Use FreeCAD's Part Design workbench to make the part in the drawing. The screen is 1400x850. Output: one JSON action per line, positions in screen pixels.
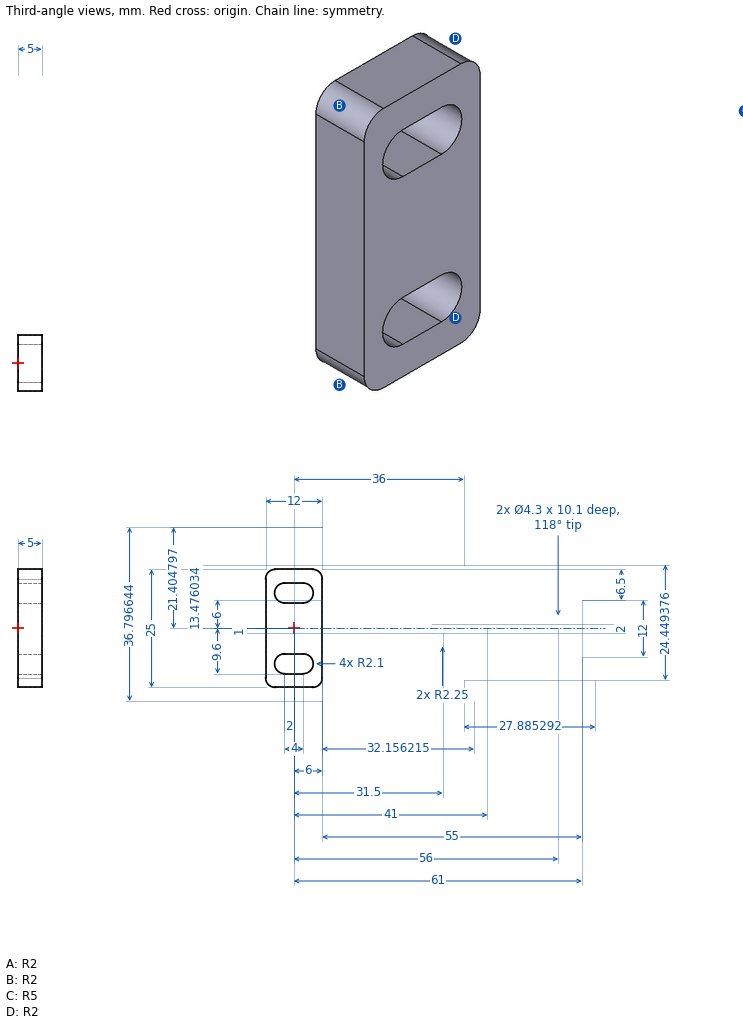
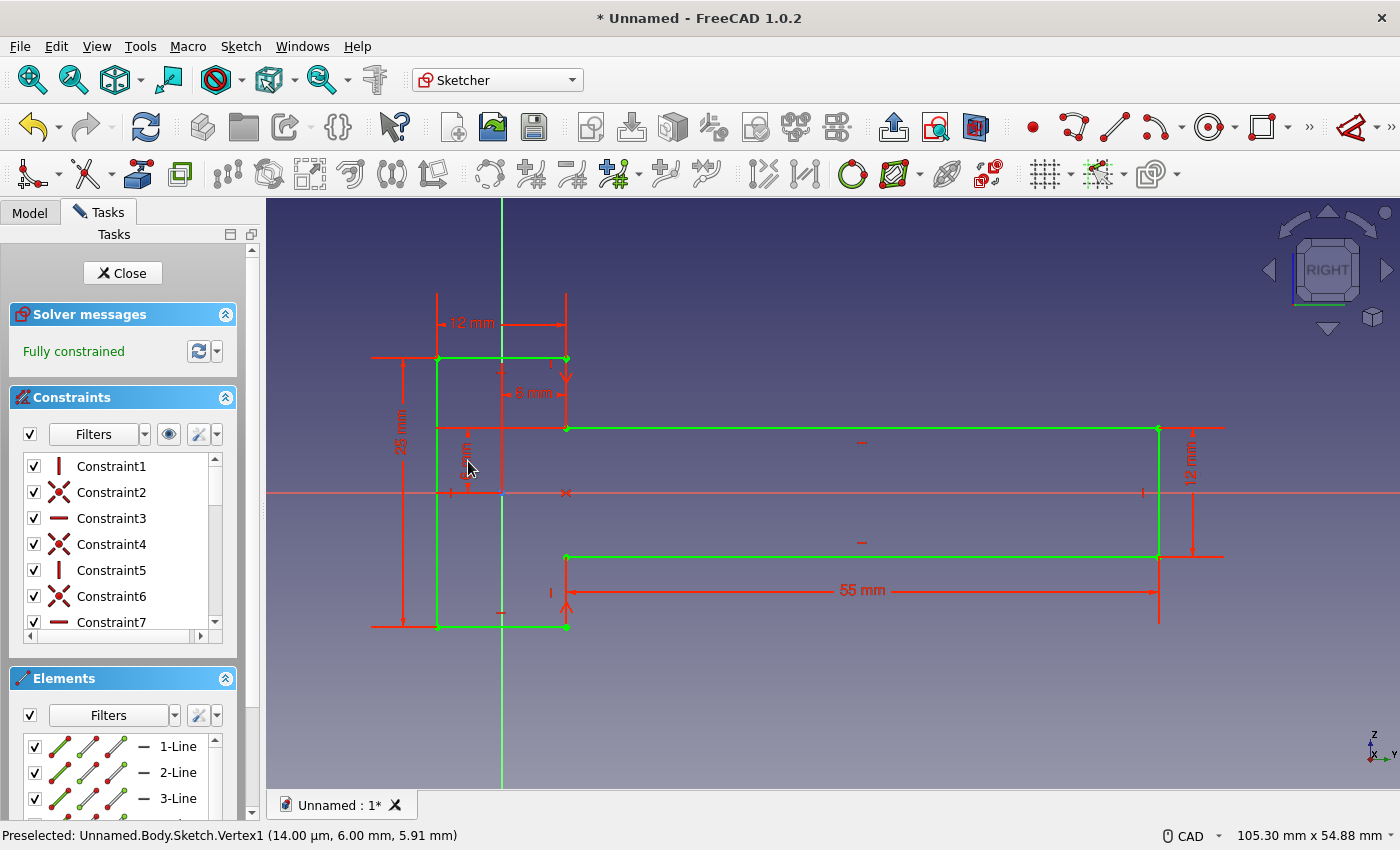
{"action": "left_click", "coordinate": [123, 273]}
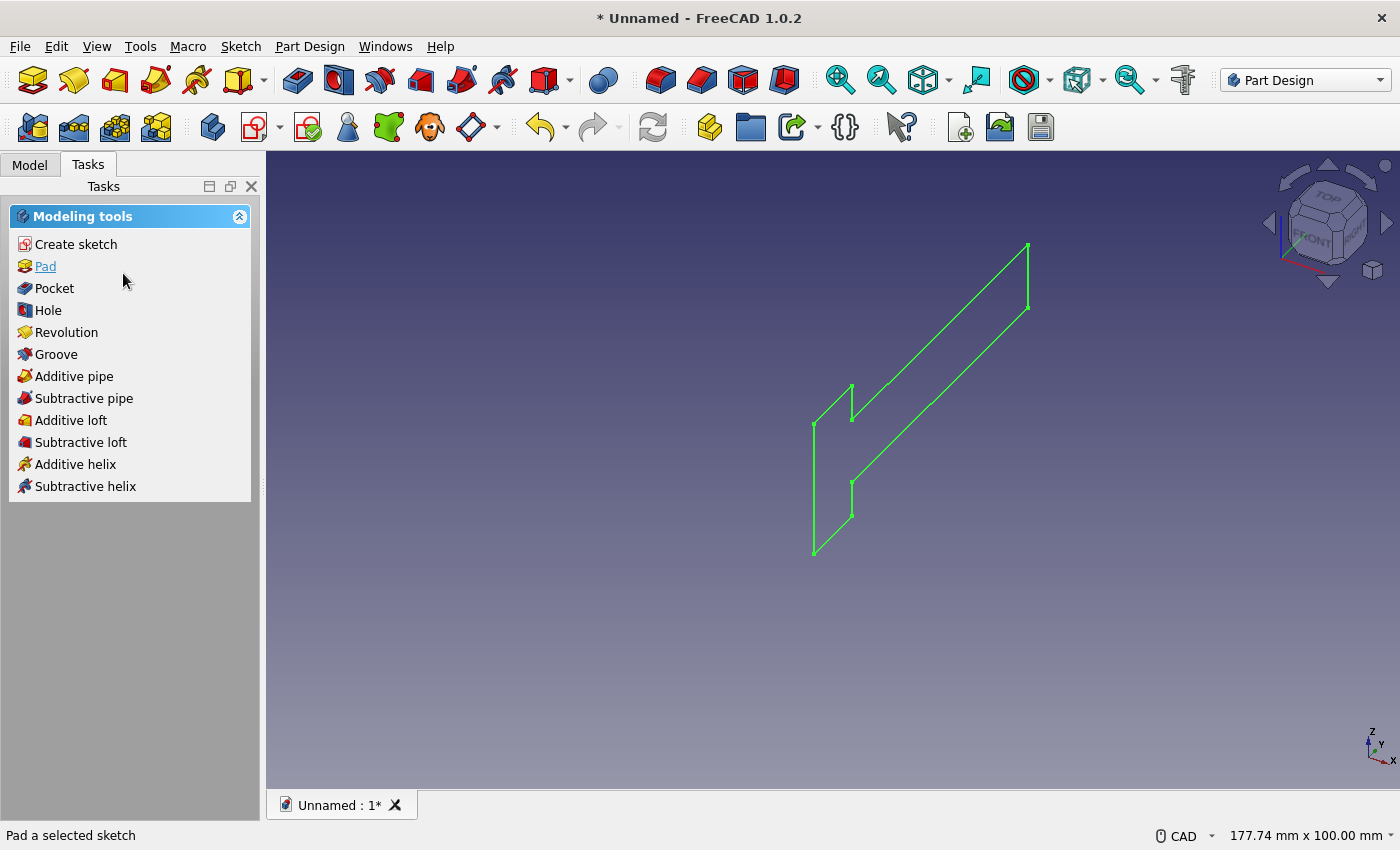
{"action": "left_click", "coordinate": [33, 80]}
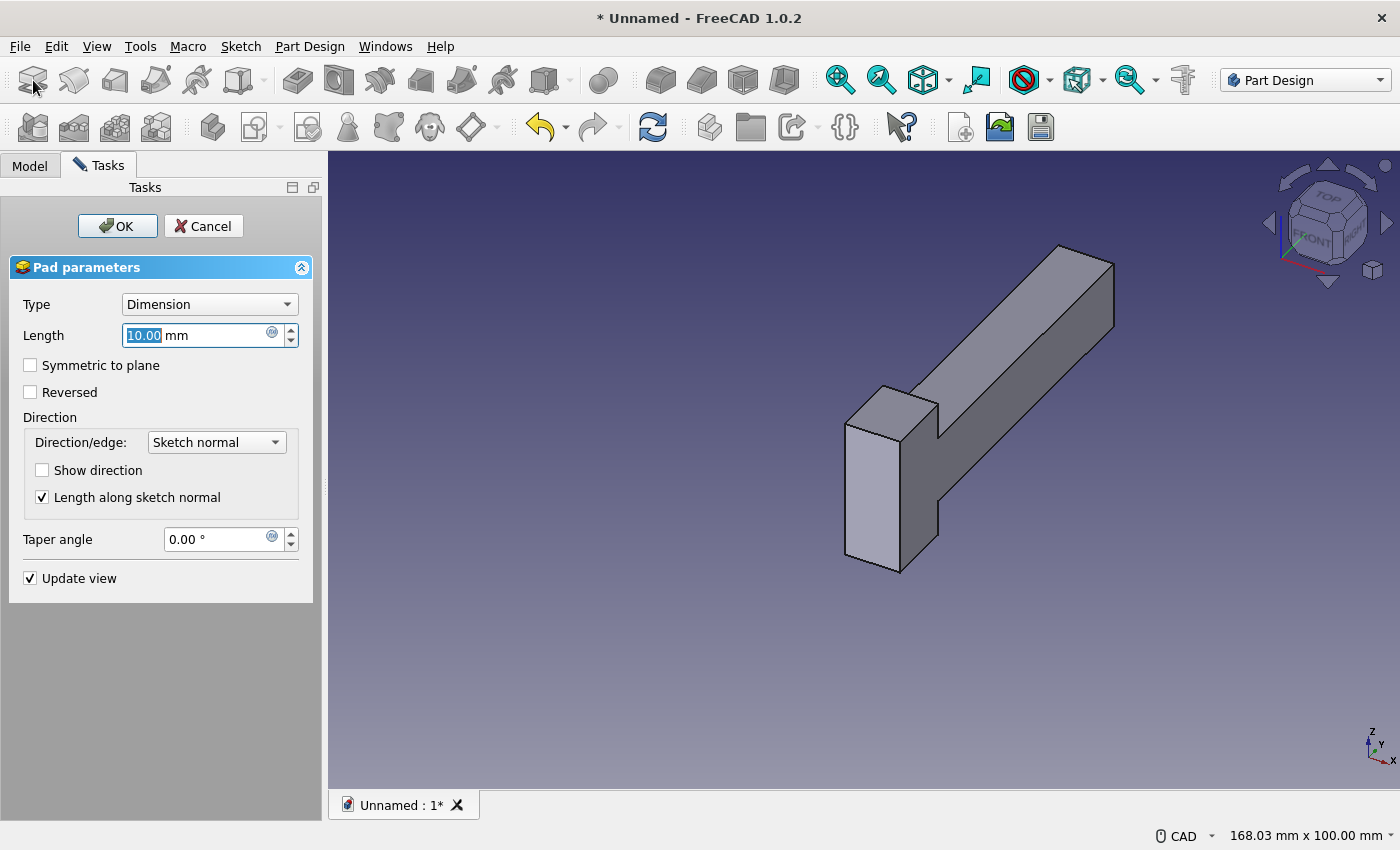
{"action": "type", "text": "5"}
{"action": "key", "text": "Tab"}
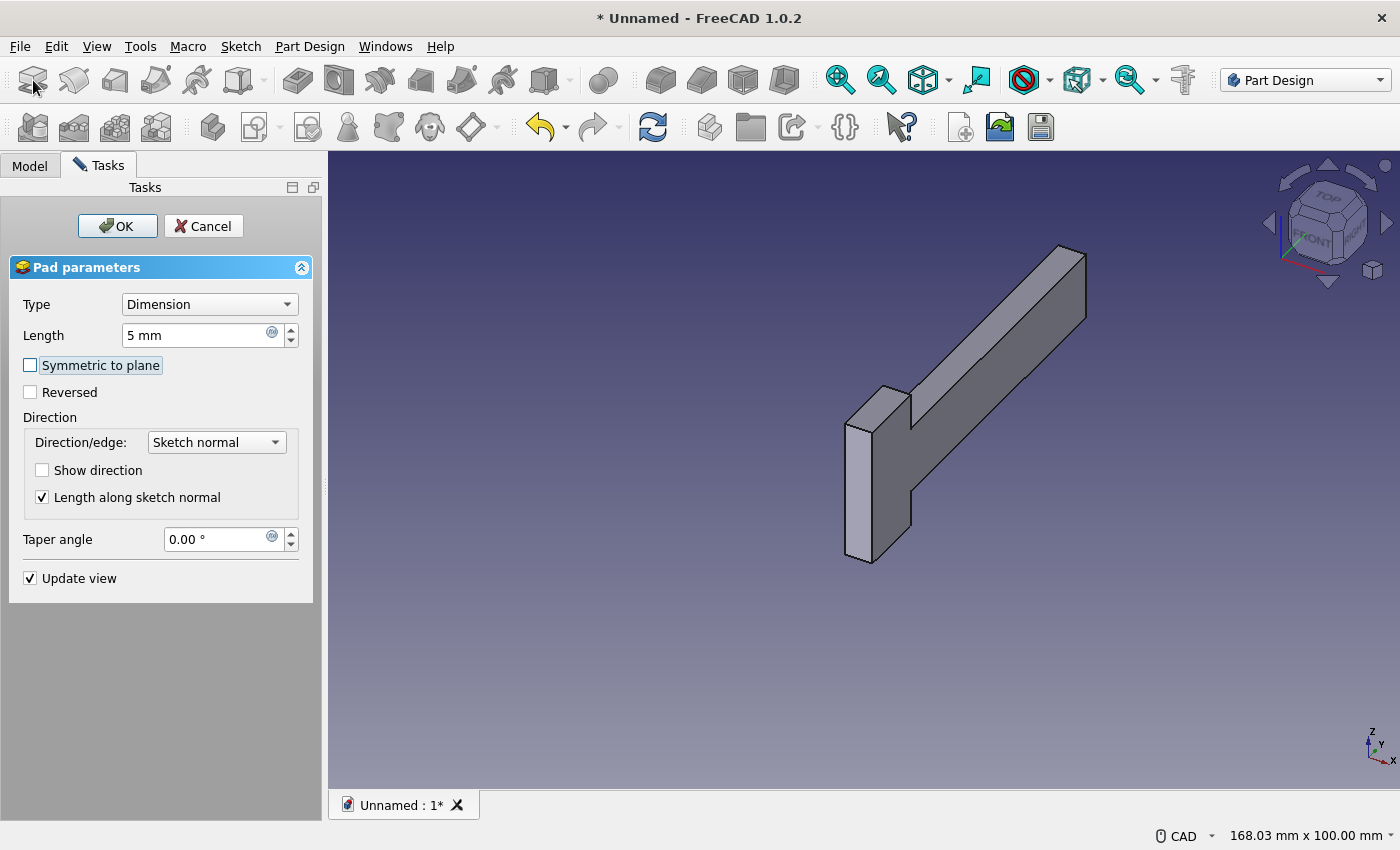
{"action": "left_click", "coordinate": [118, 226]}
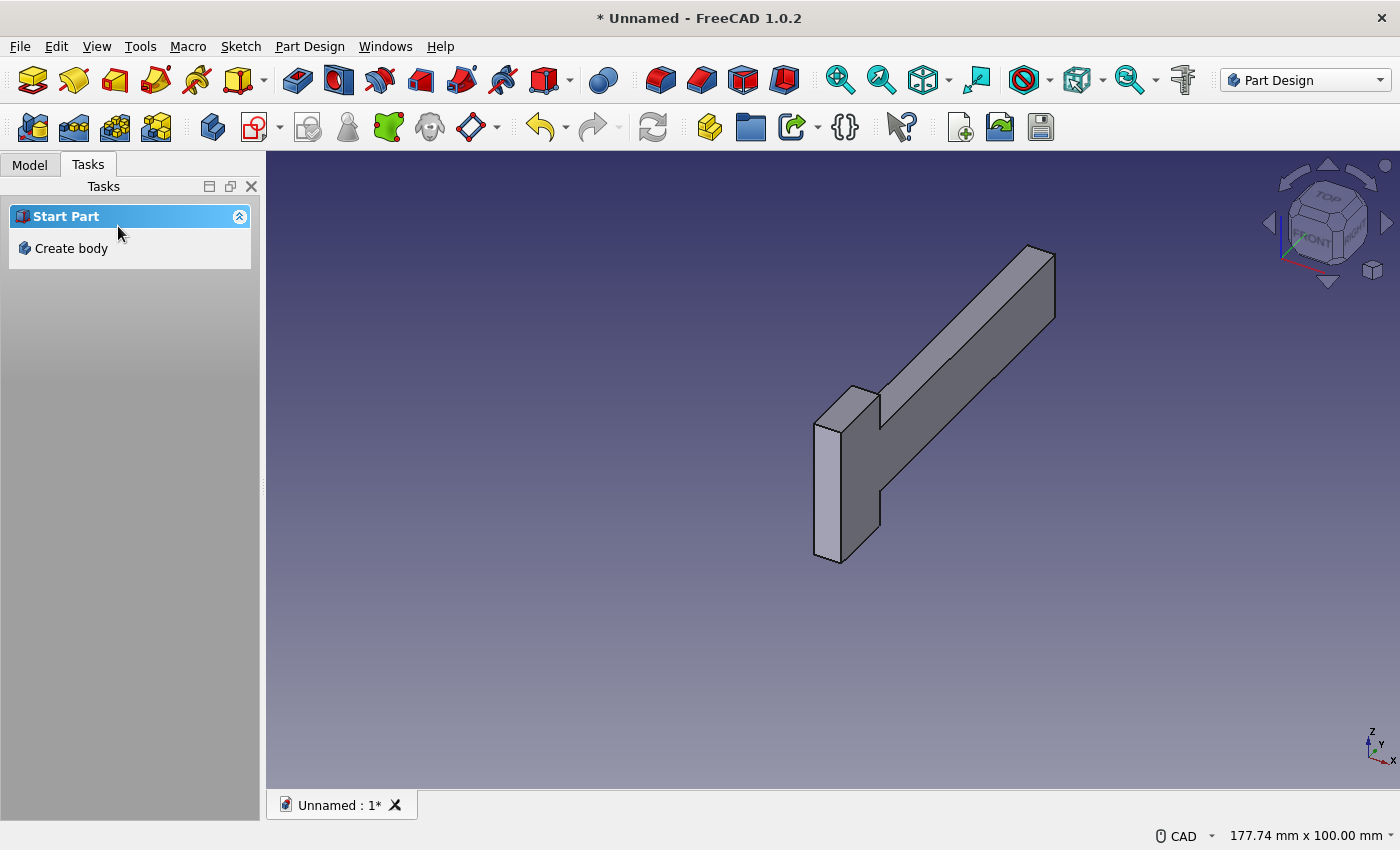
{"action": "key", "text": "6"}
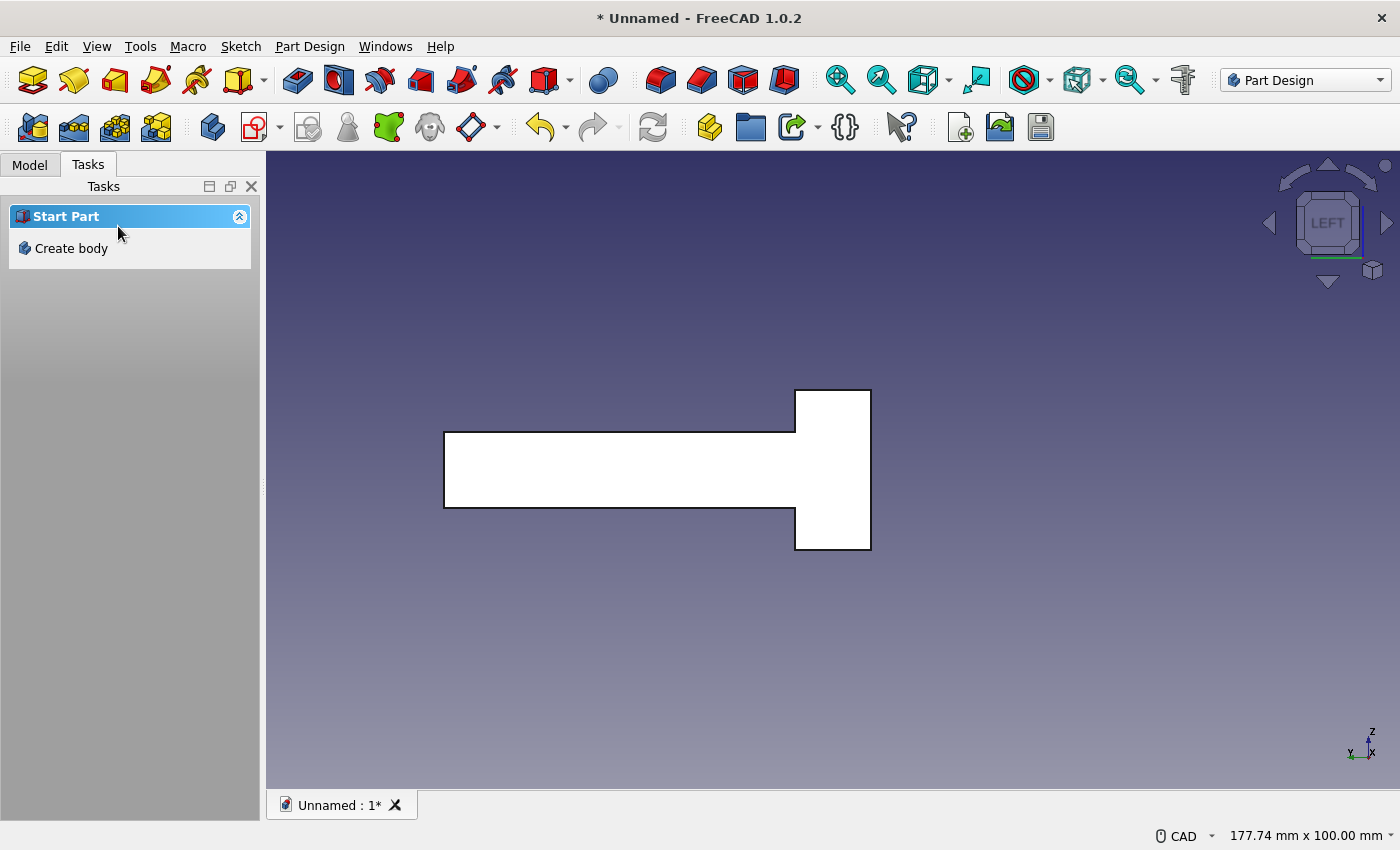
{"action": "left_click", "coordinate": [841, 80]}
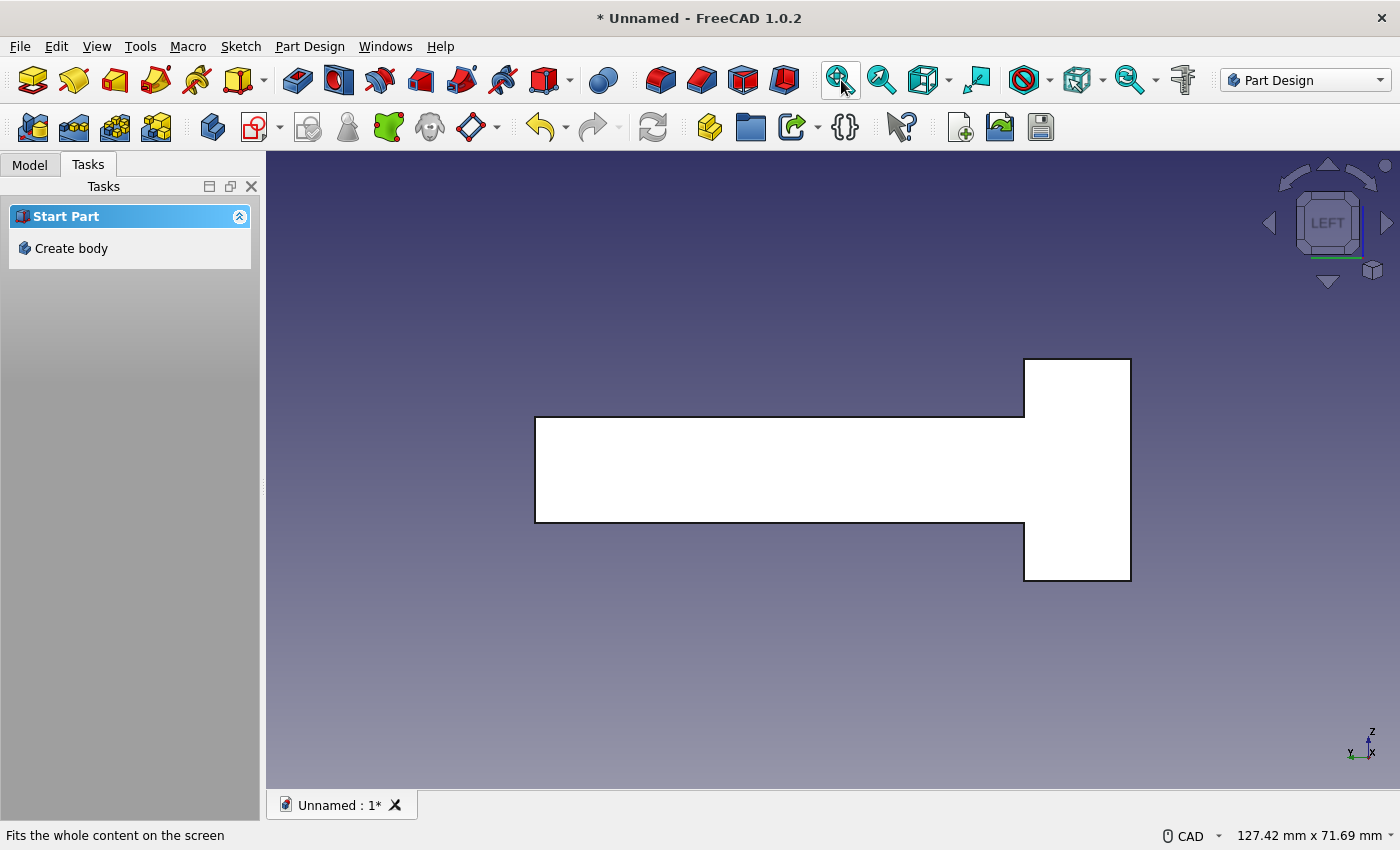
{"action": "left_click", "coordinate": [748, 469]}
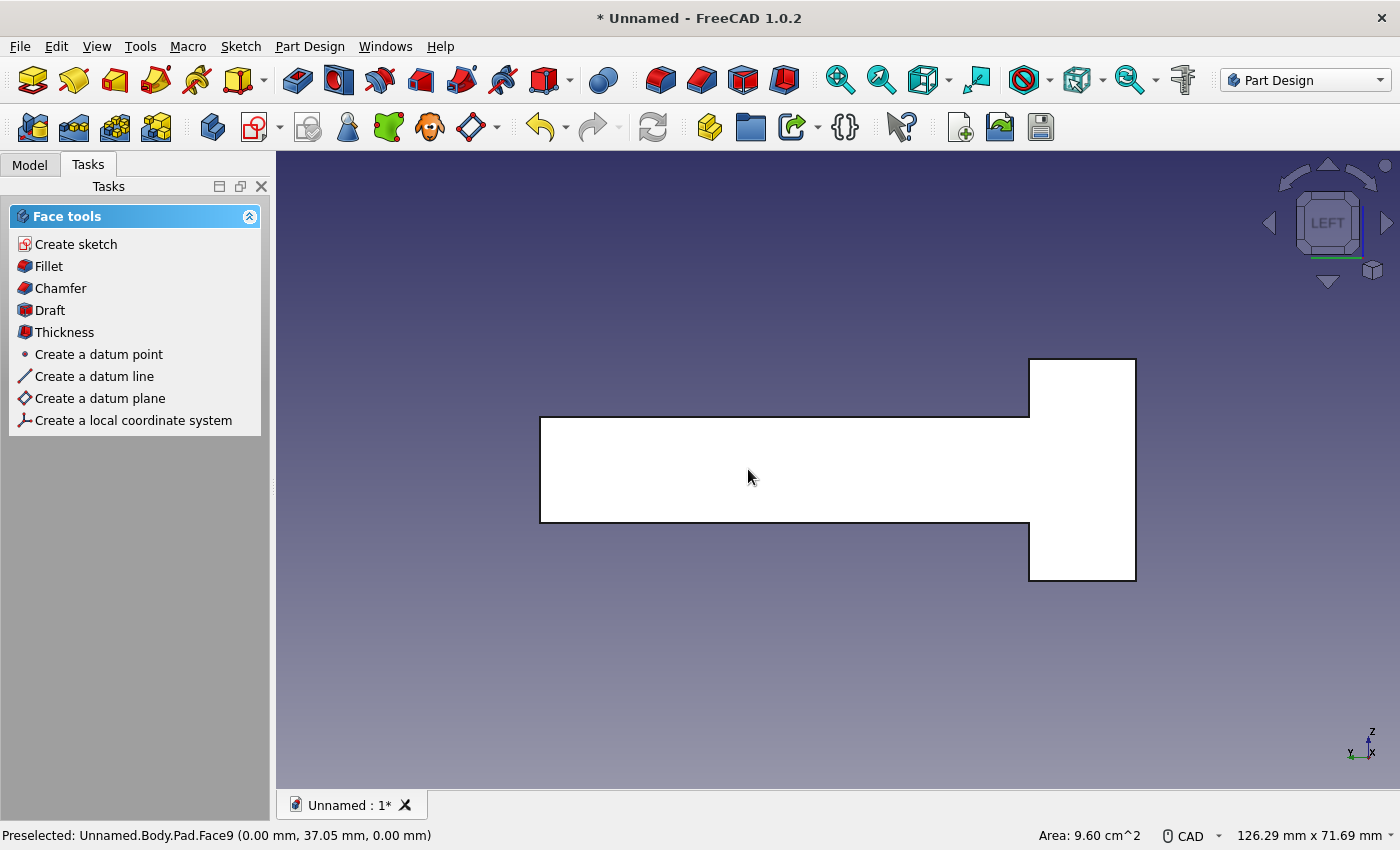
{"action": "left_click", "coordinate": [254, 128]}